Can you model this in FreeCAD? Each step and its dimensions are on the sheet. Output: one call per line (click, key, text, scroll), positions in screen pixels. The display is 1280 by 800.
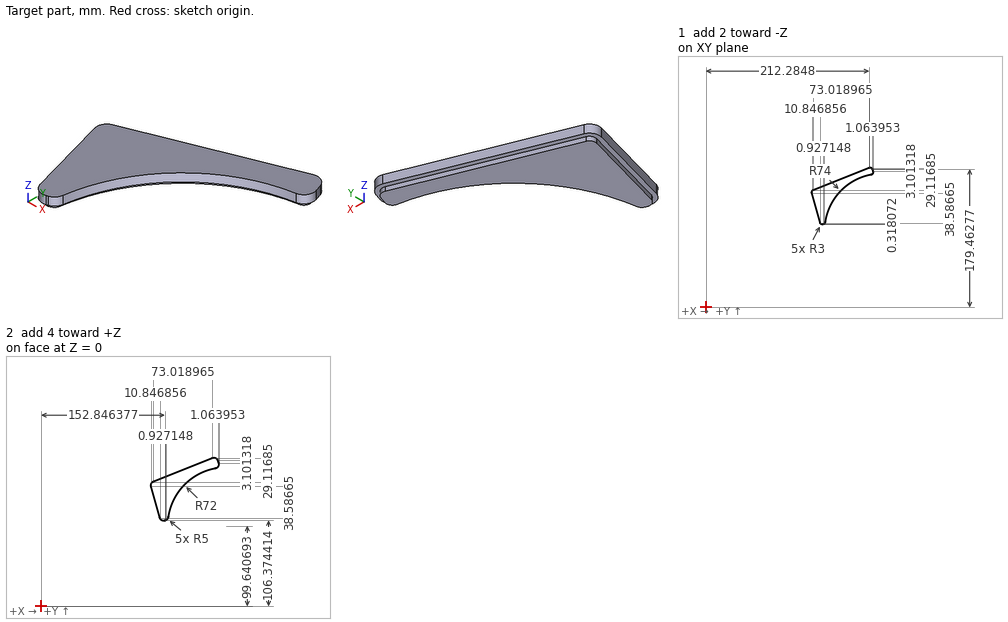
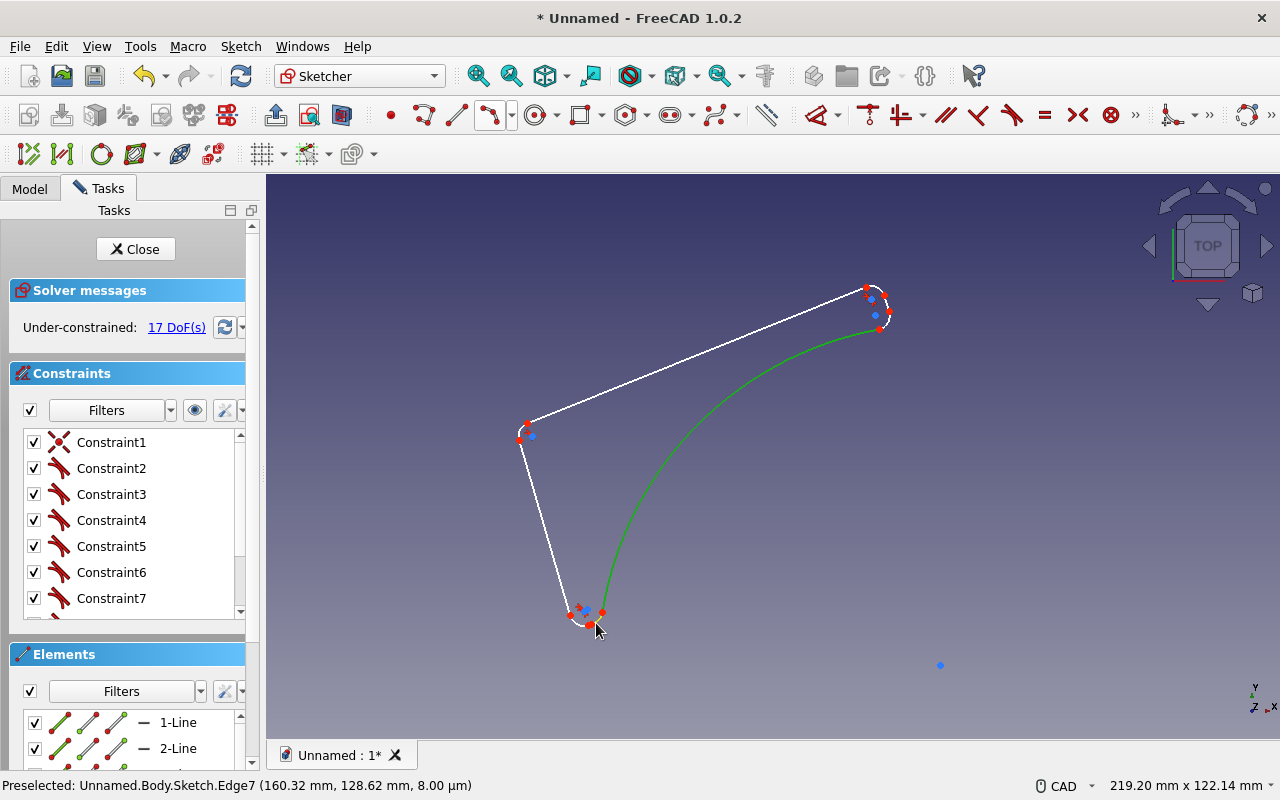
scroll(885, 326, up, 4)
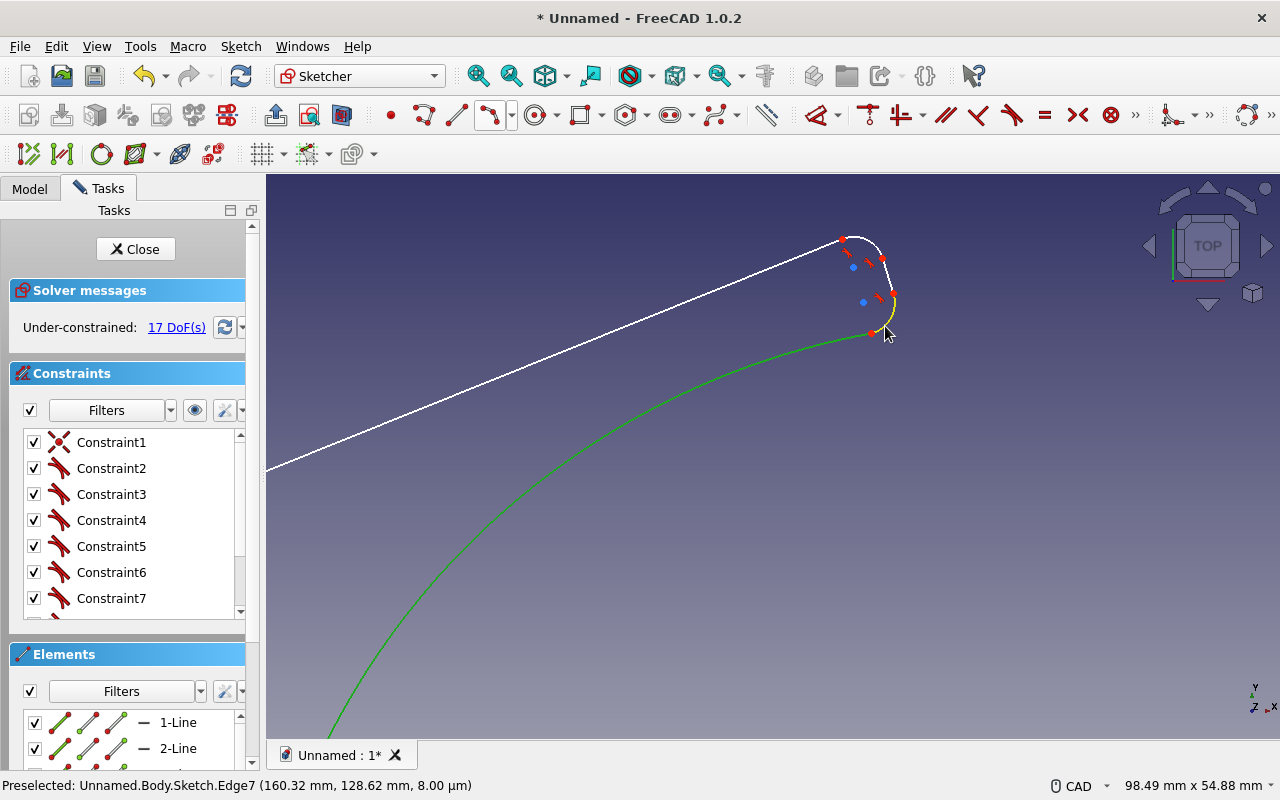
click(885, 326)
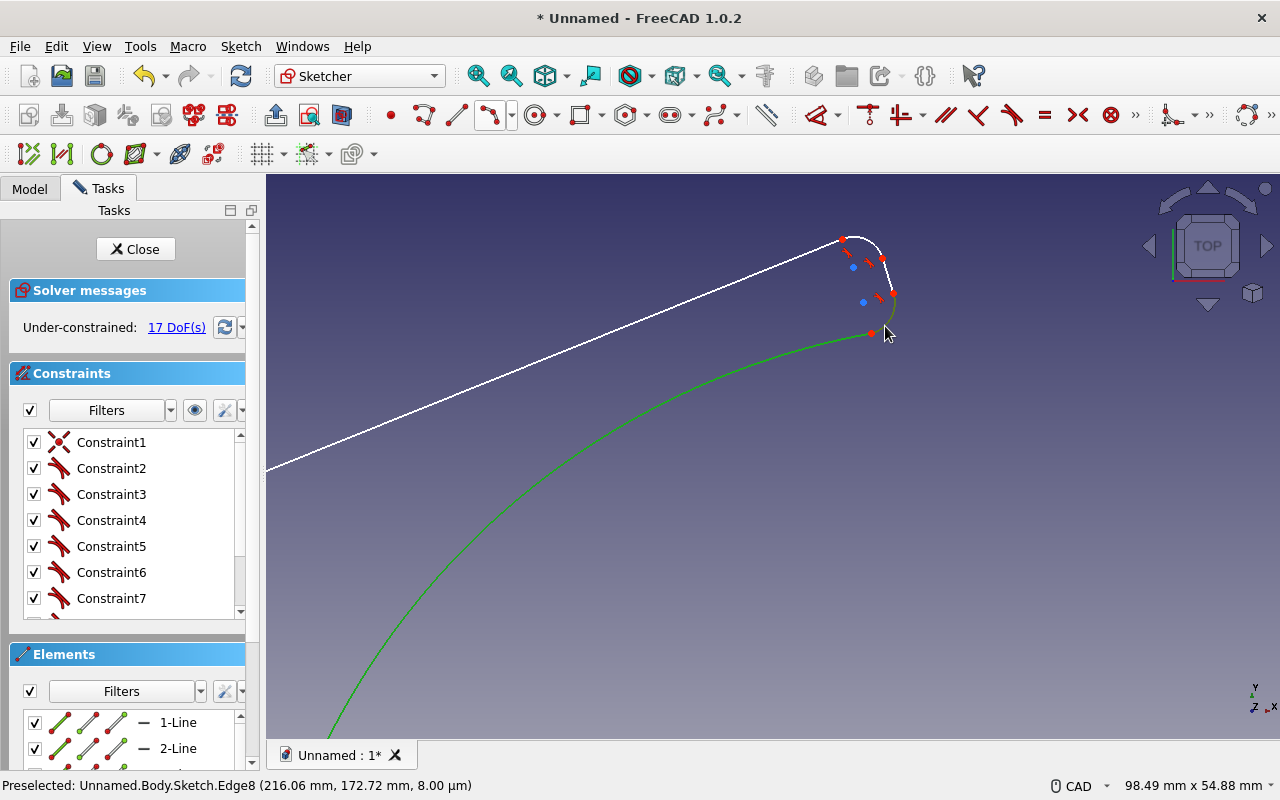
click(1012, 116)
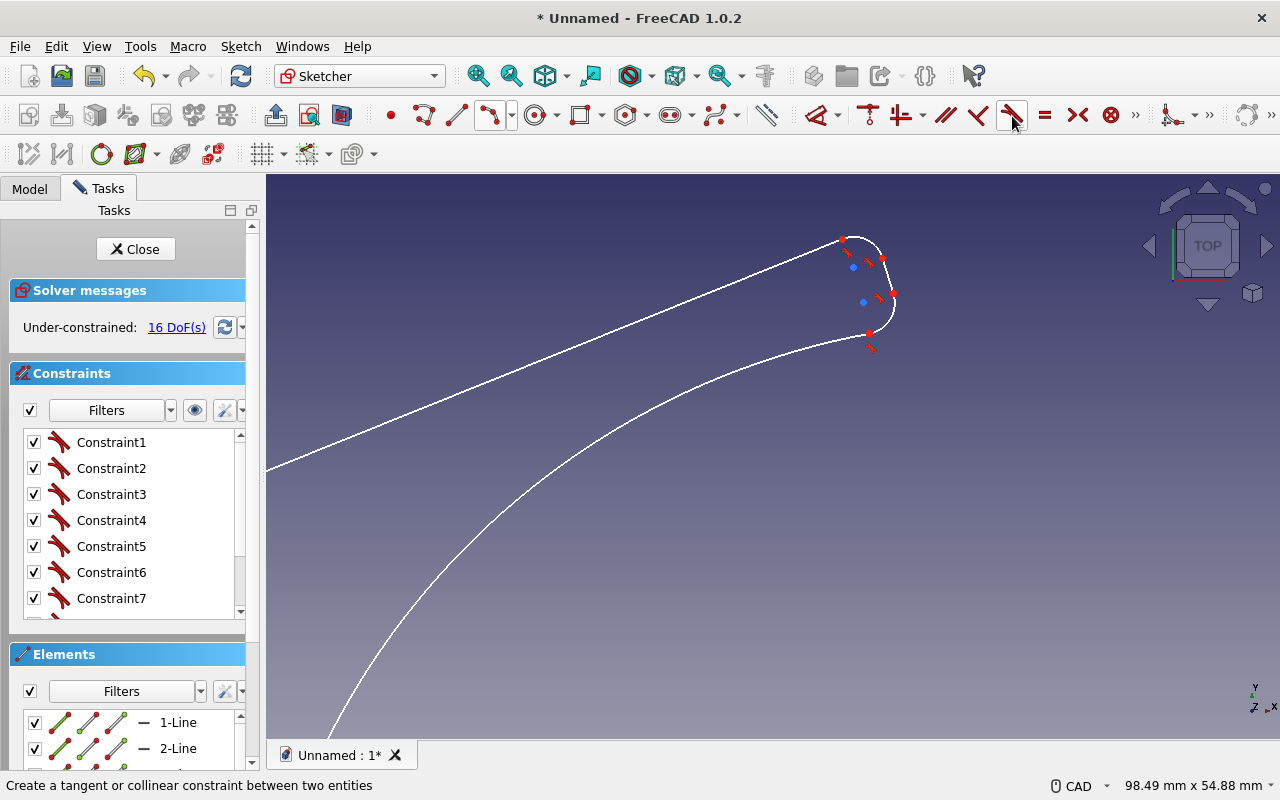
scroll(885, 325, down, 4)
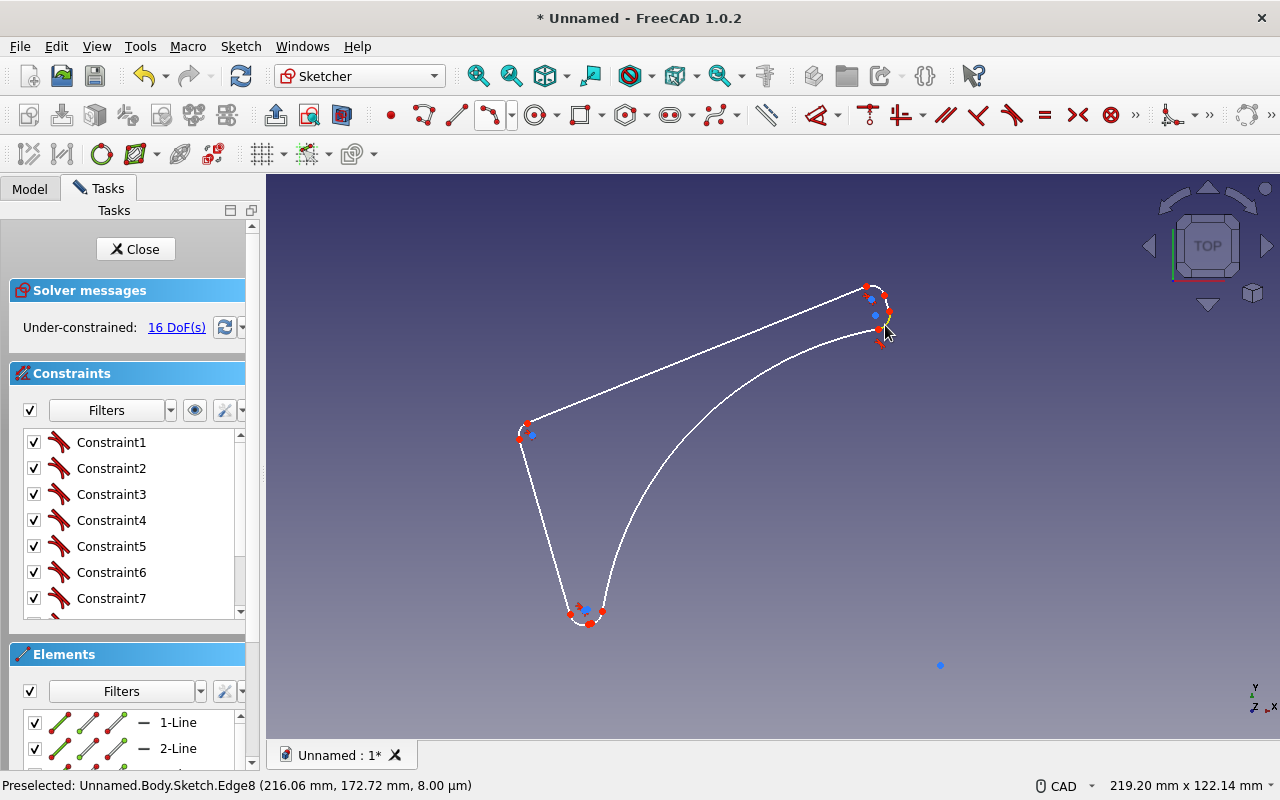
scroll(574, 621, up, 4)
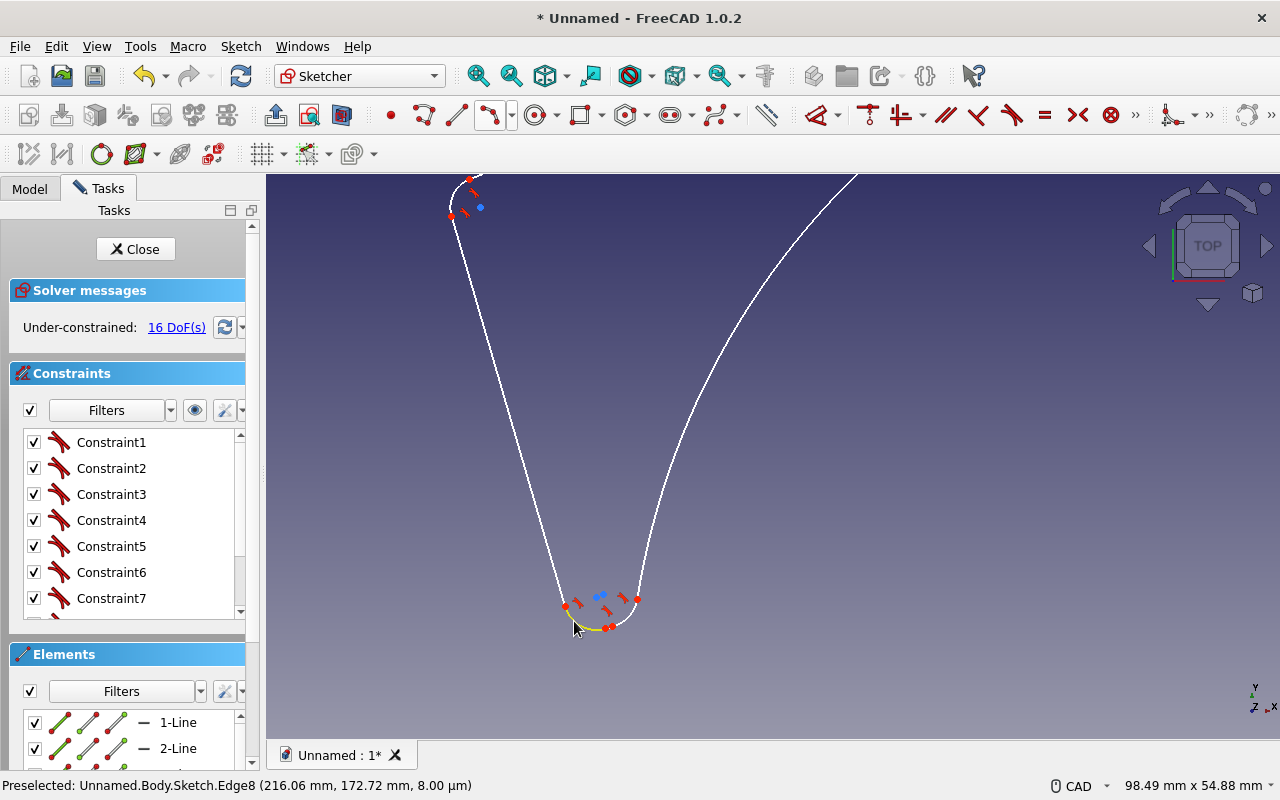
click(573, 620)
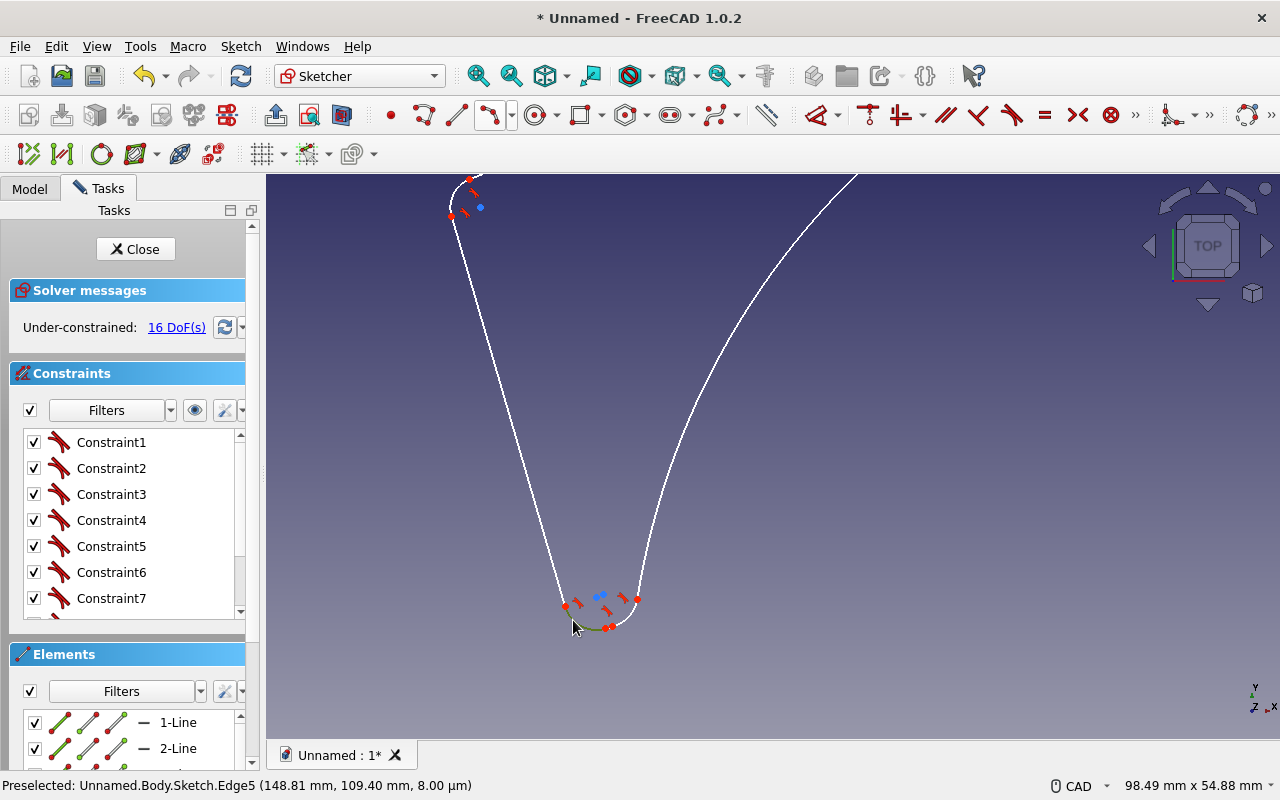
click(623, 622)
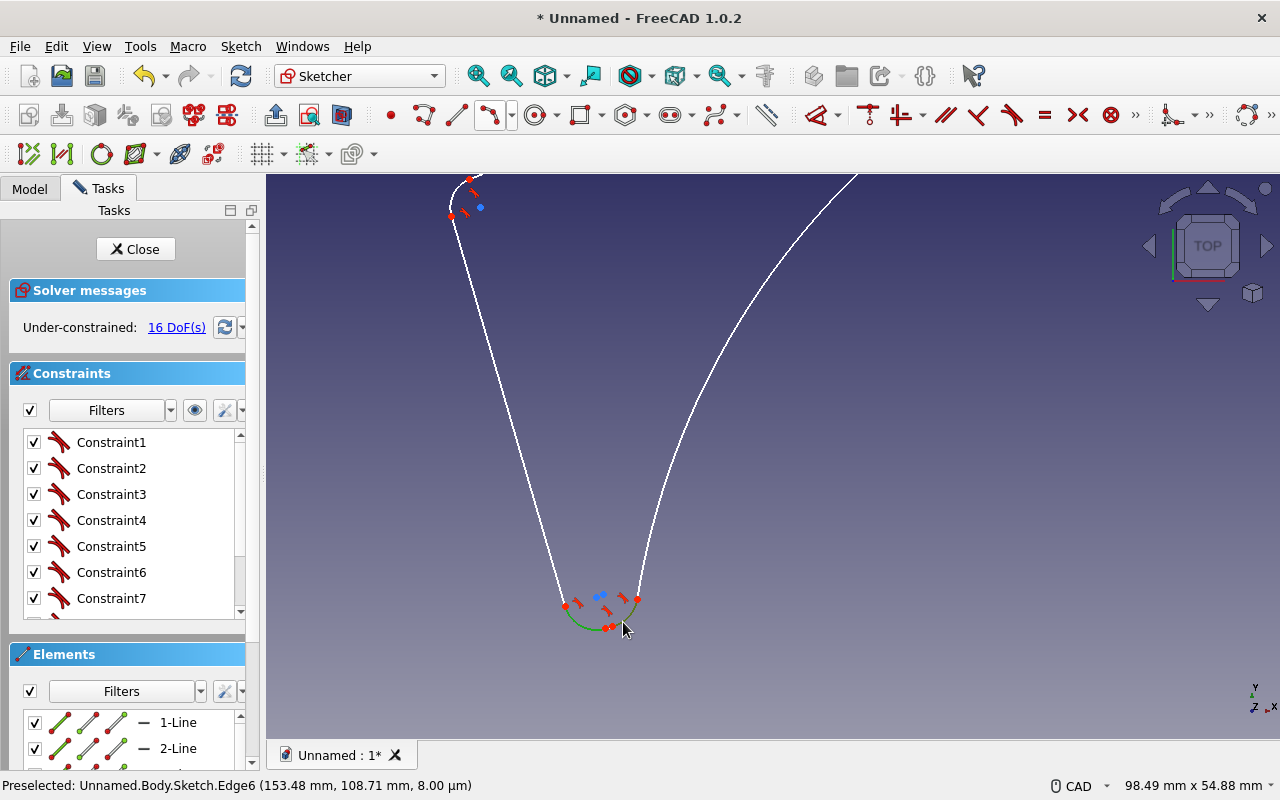
scroll(574, 621, down, 4)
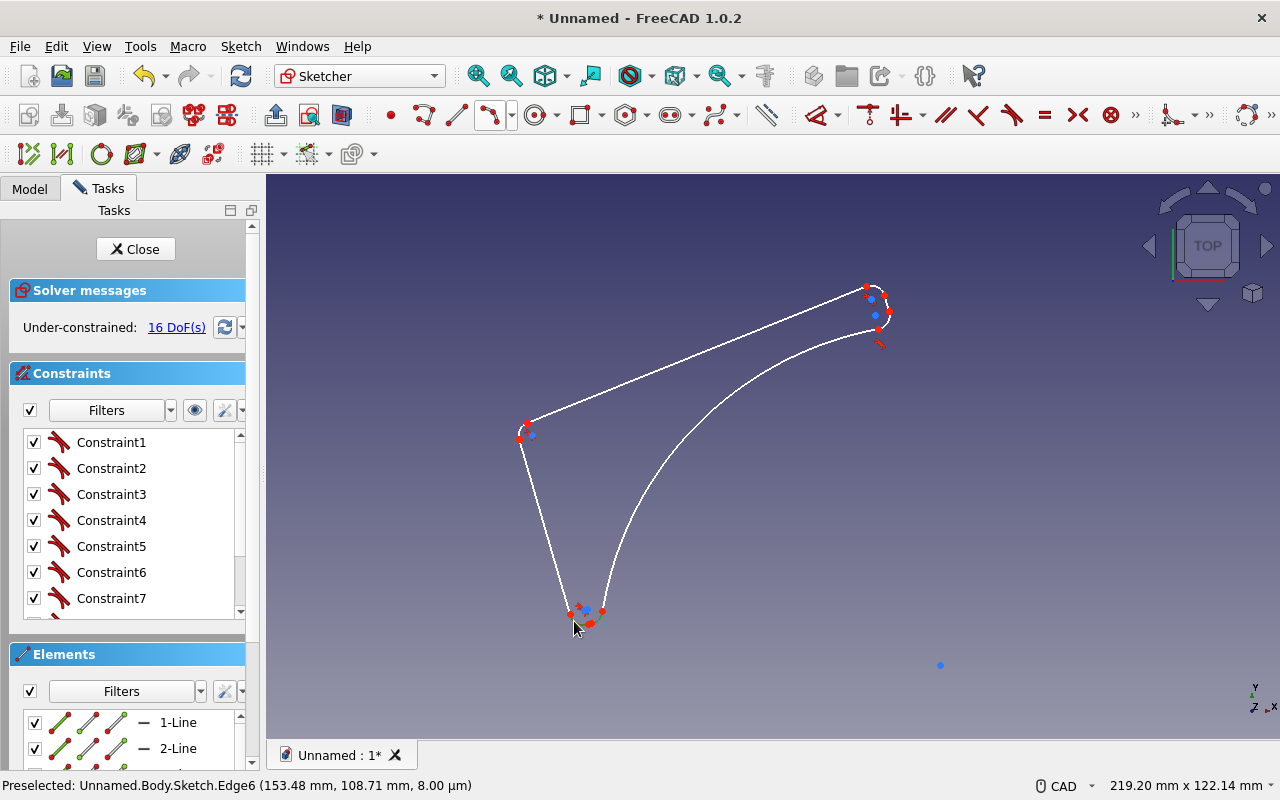
scroll(885, 326, up, 4)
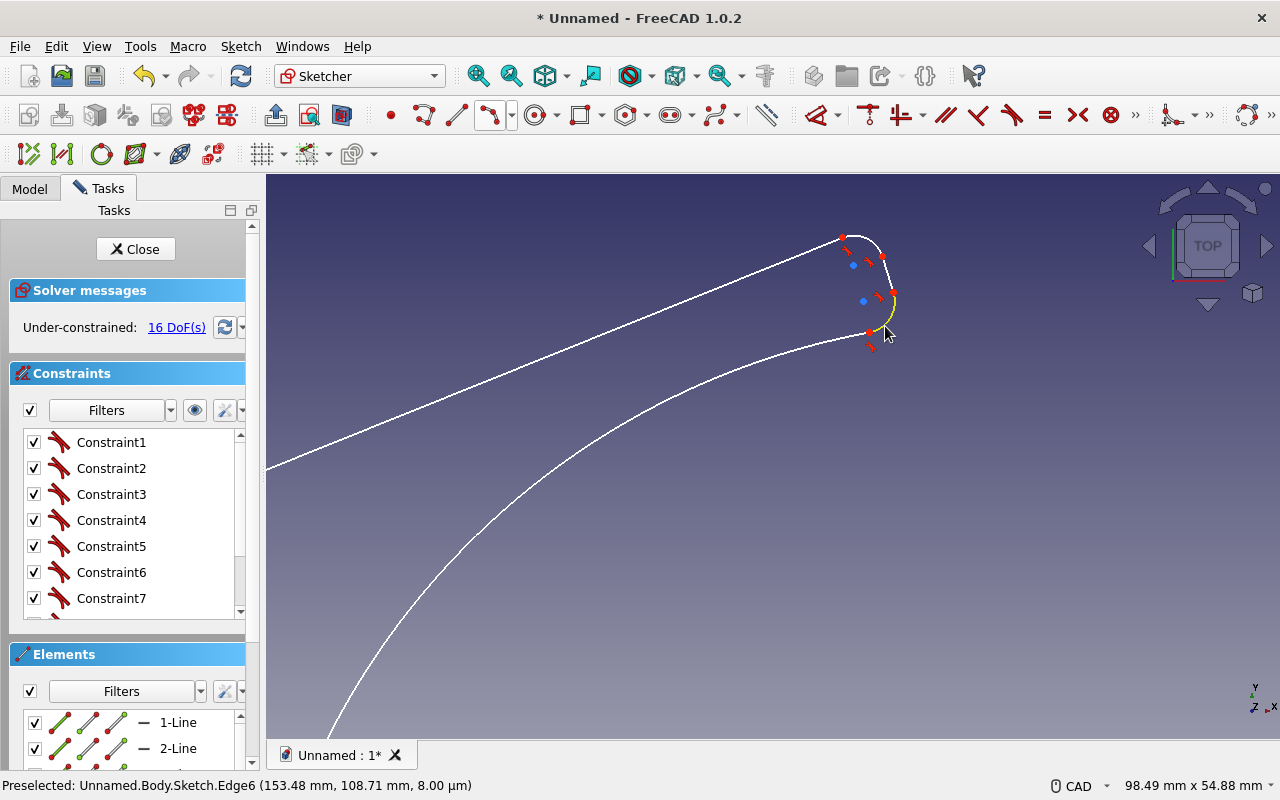
click(883, 326)